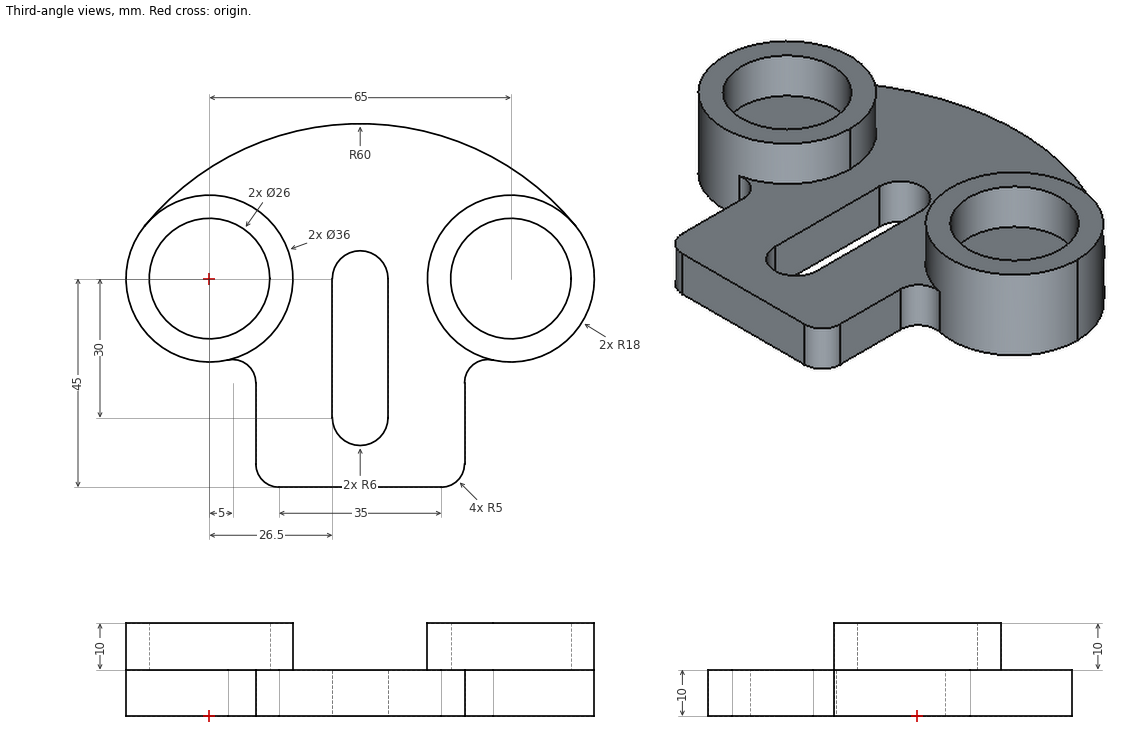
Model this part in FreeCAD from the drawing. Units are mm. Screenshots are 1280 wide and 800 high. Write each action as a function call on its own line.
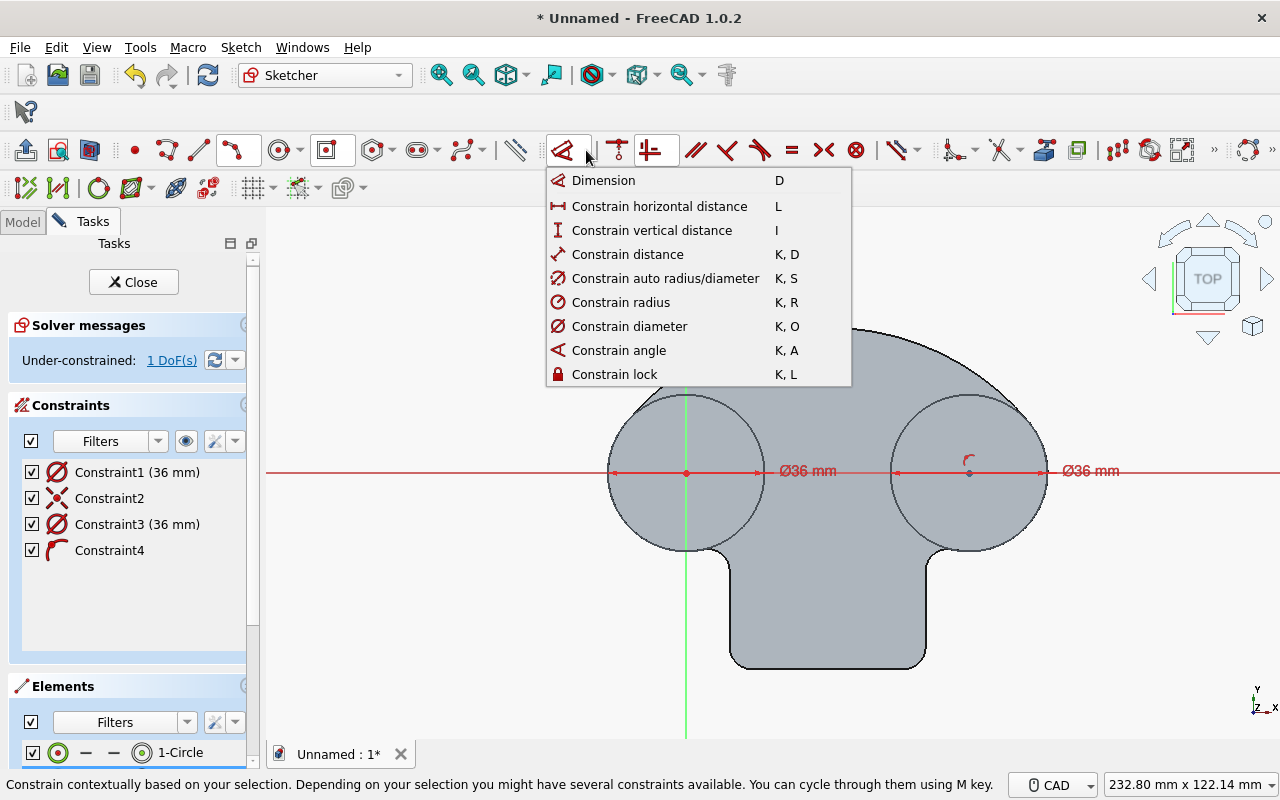
click(699, 206)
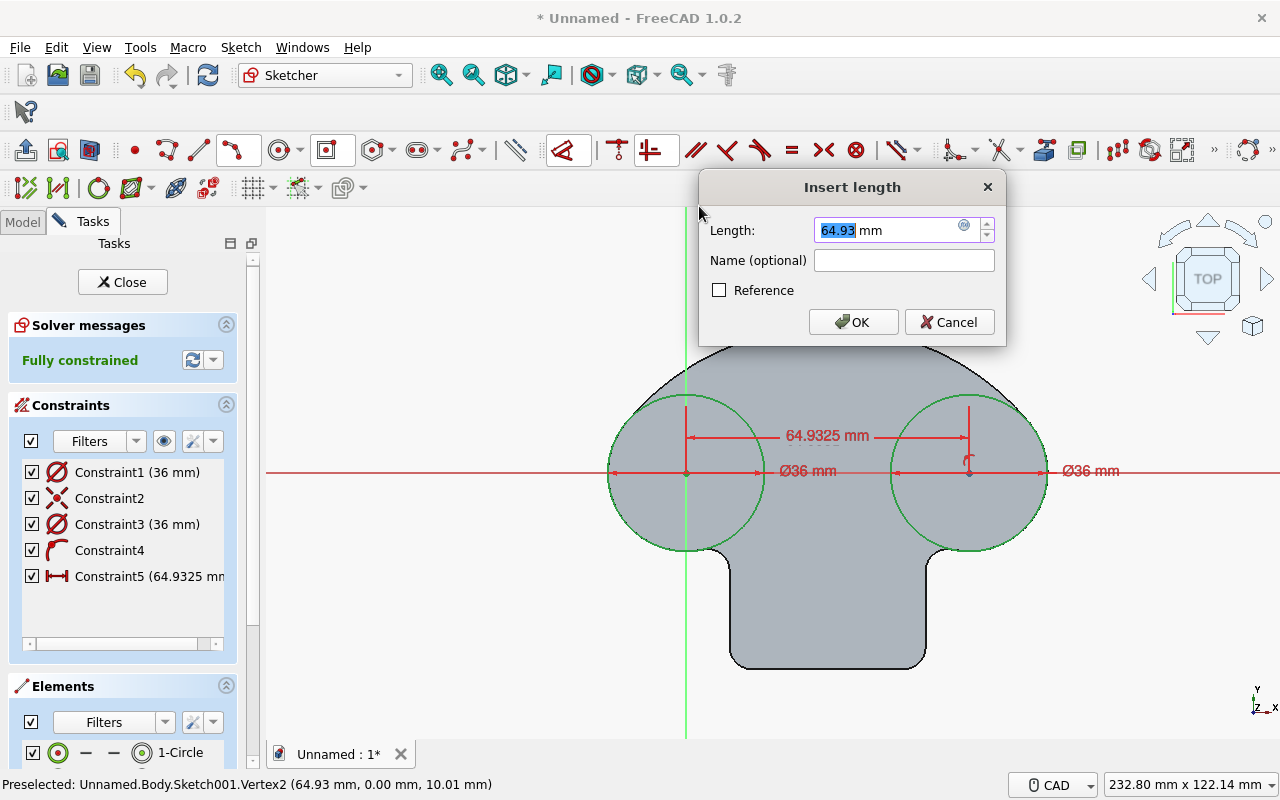
text(65)
key(Return)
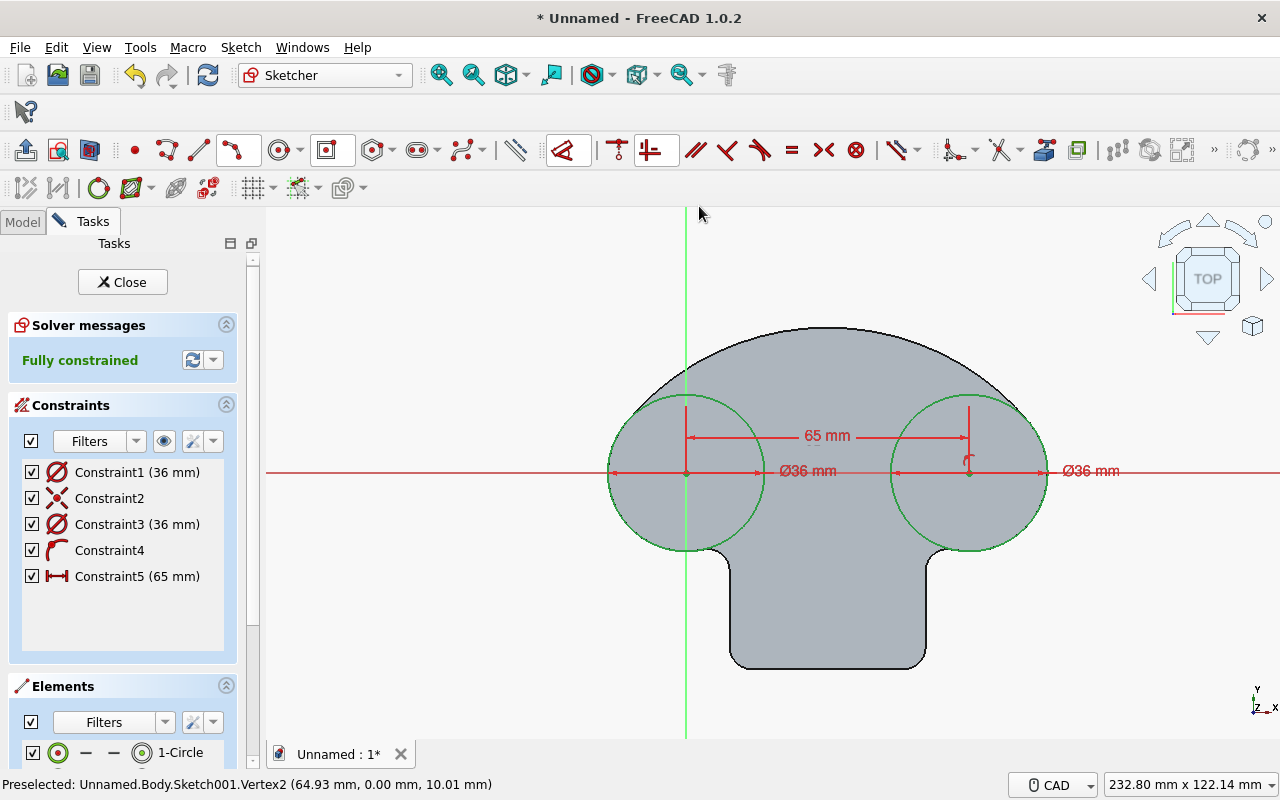
click(123, 282)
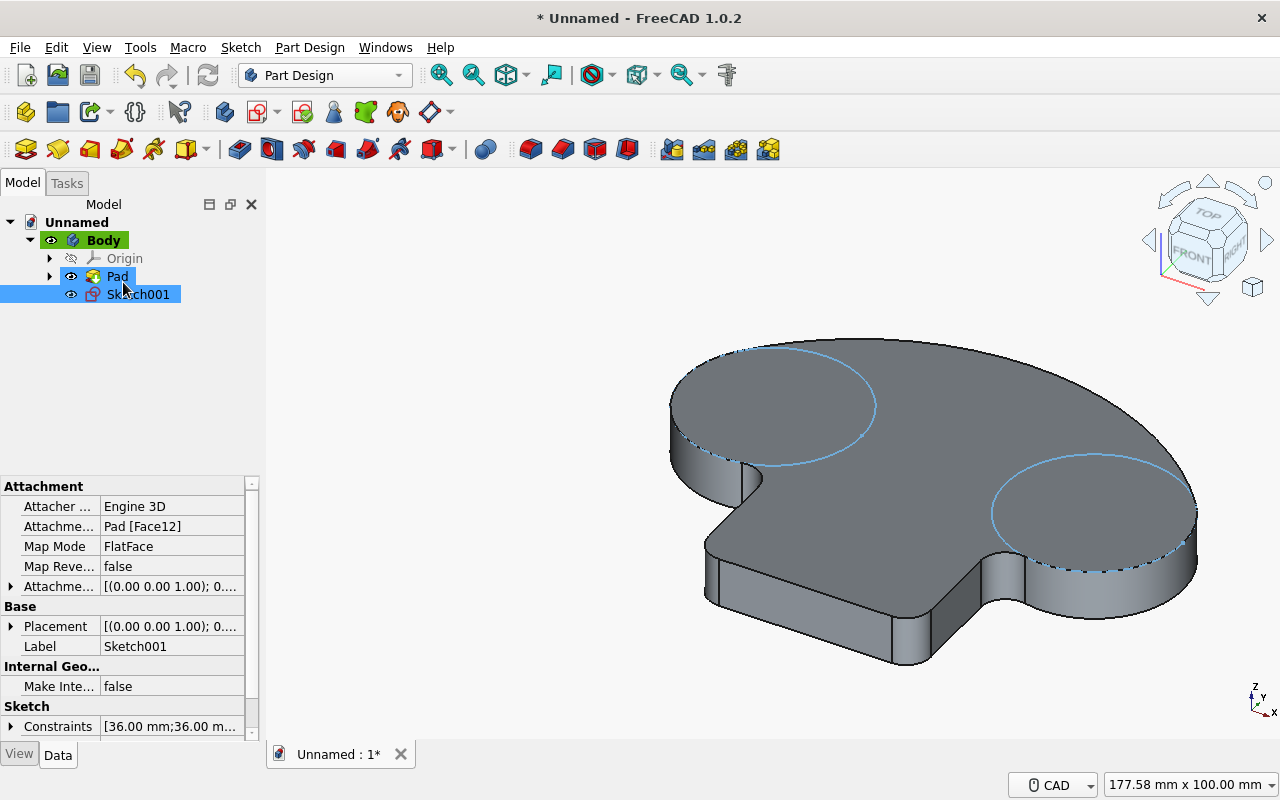
click(26, 150)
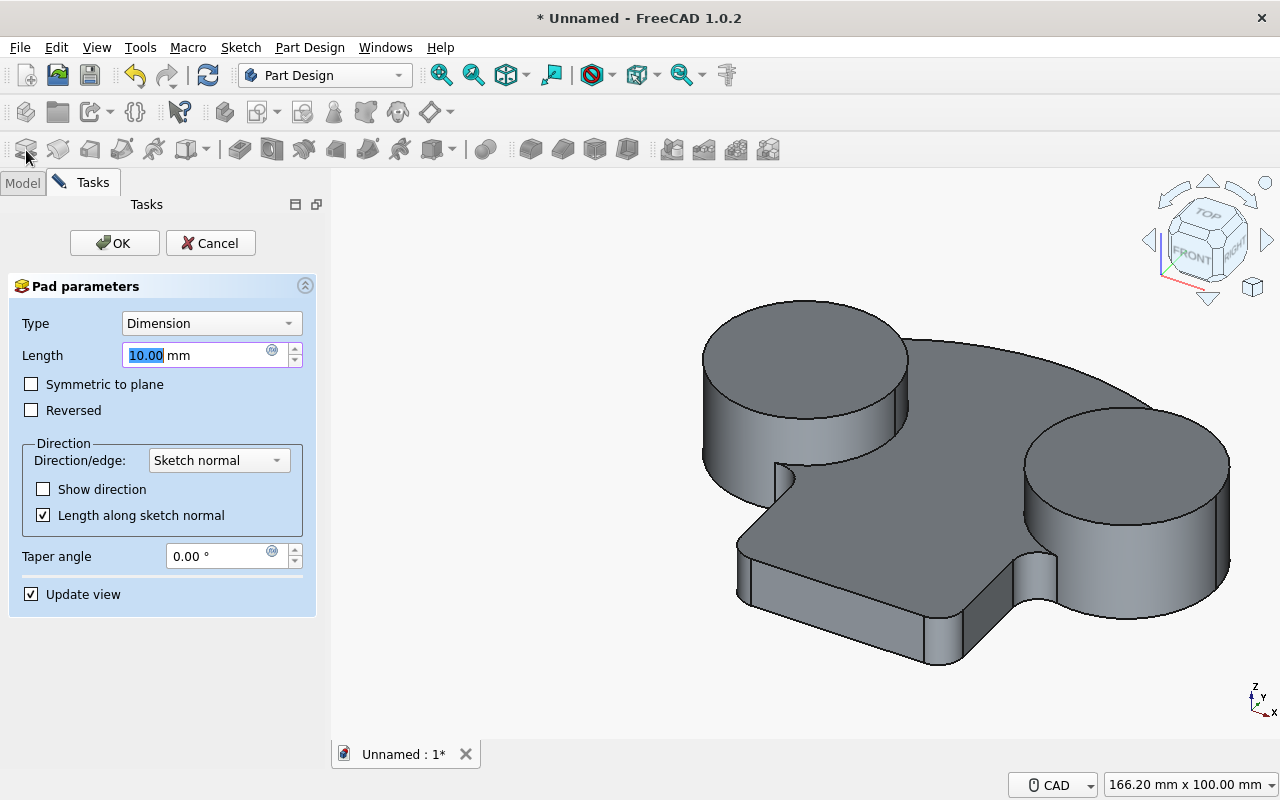
text(10)
key(Tab)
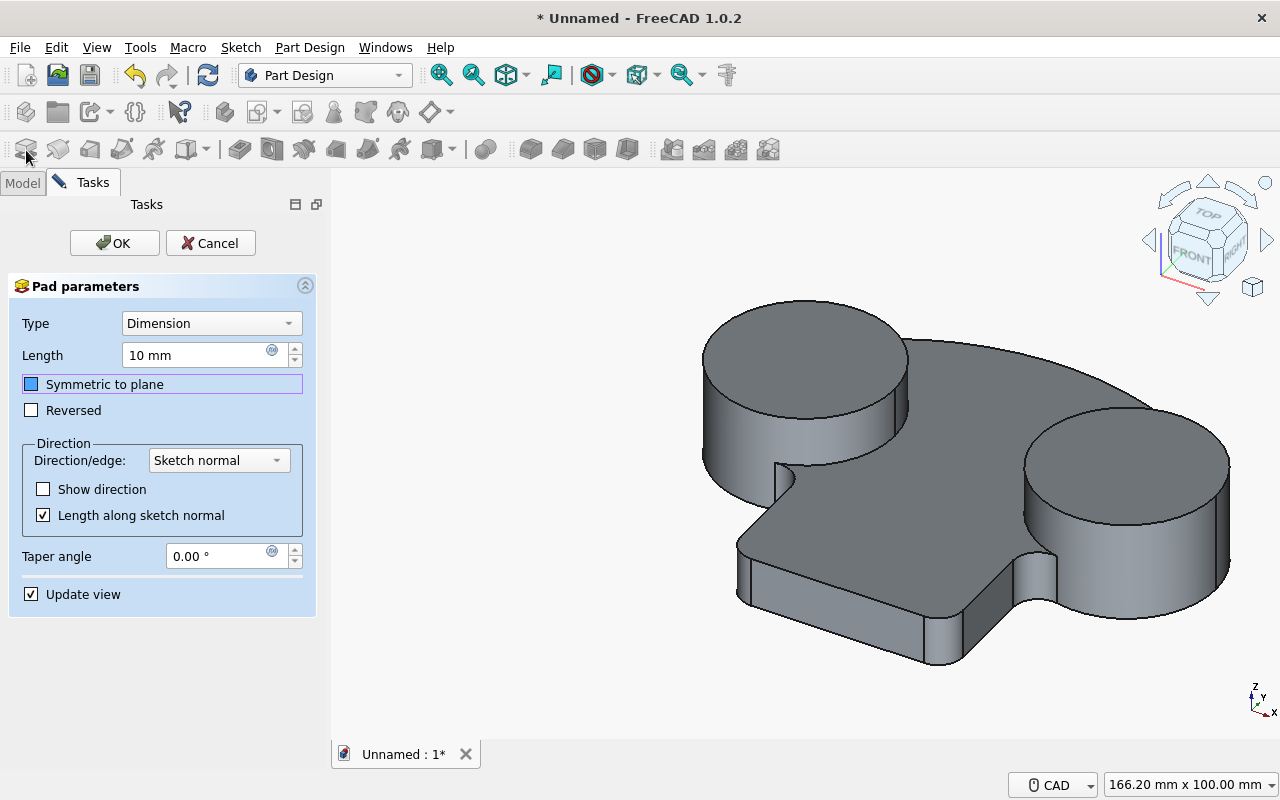
click(115, 243)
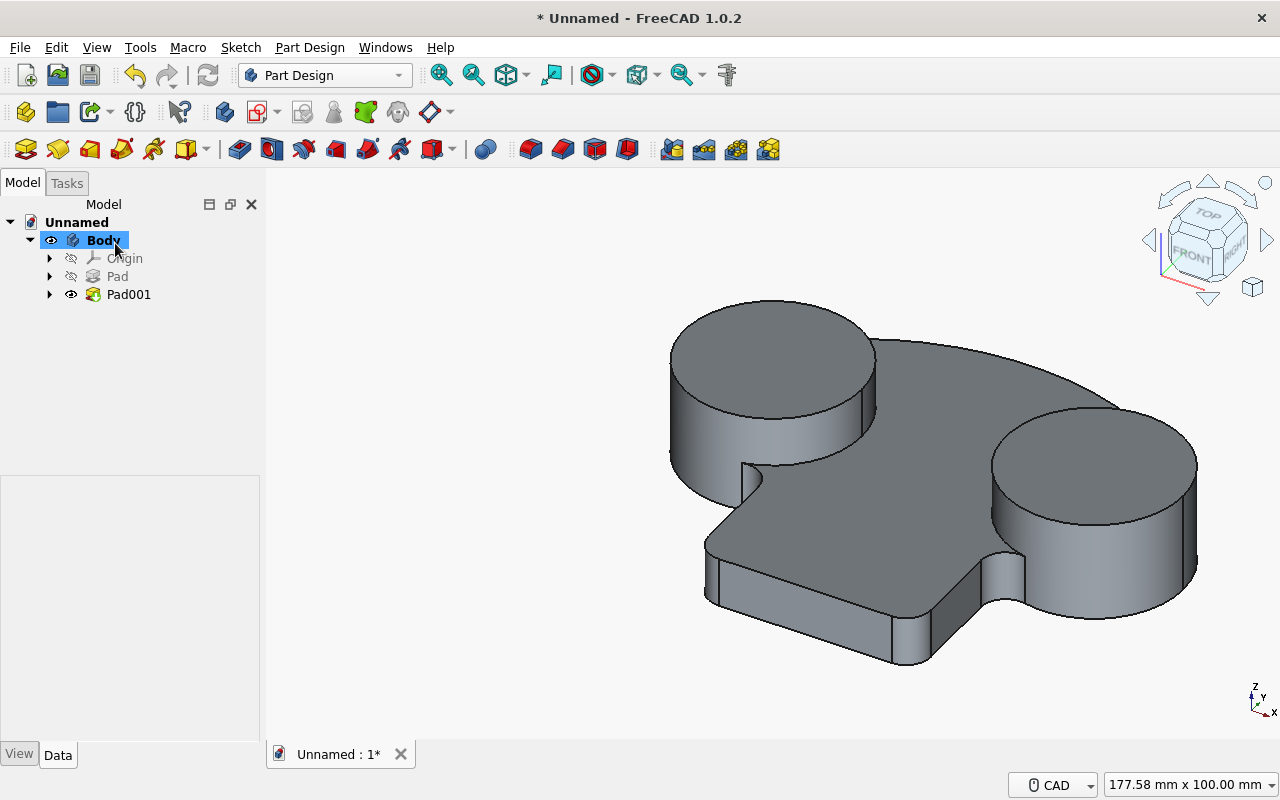
click(1094, 465)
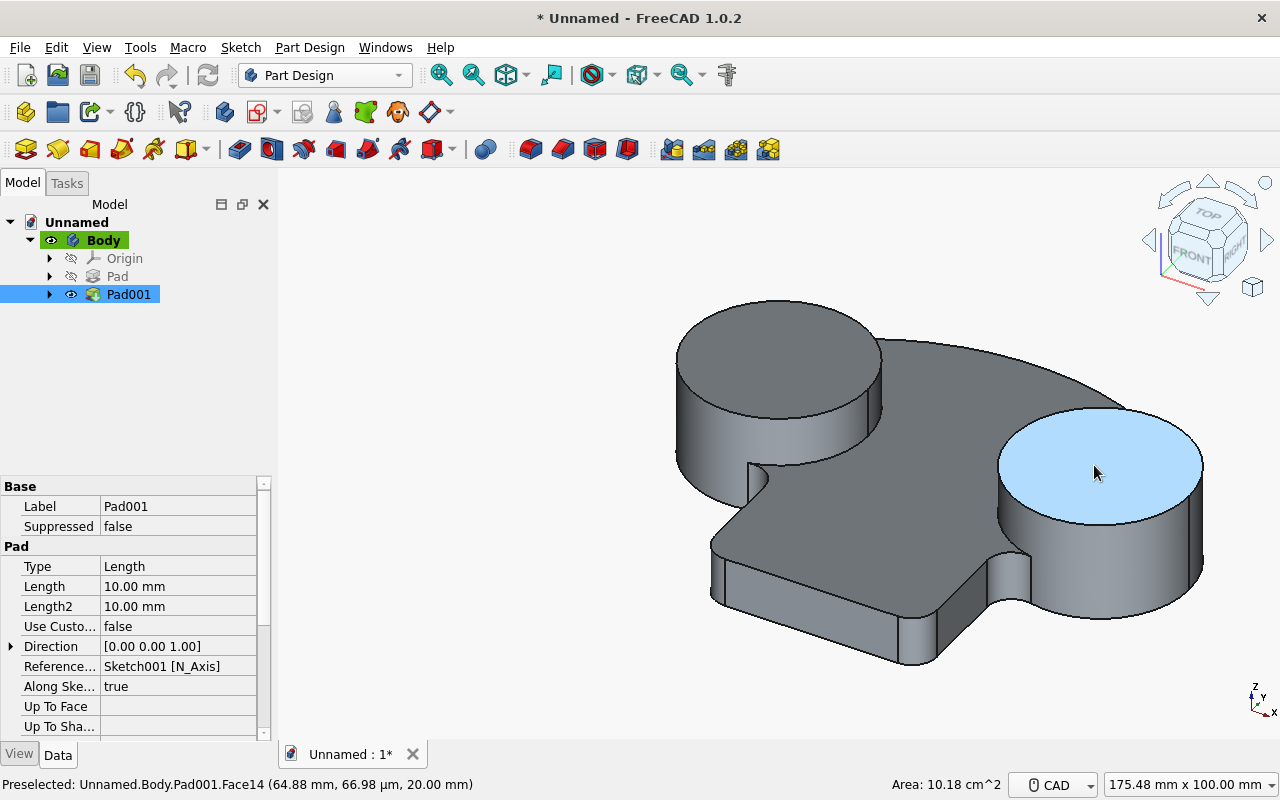
click(258, 112)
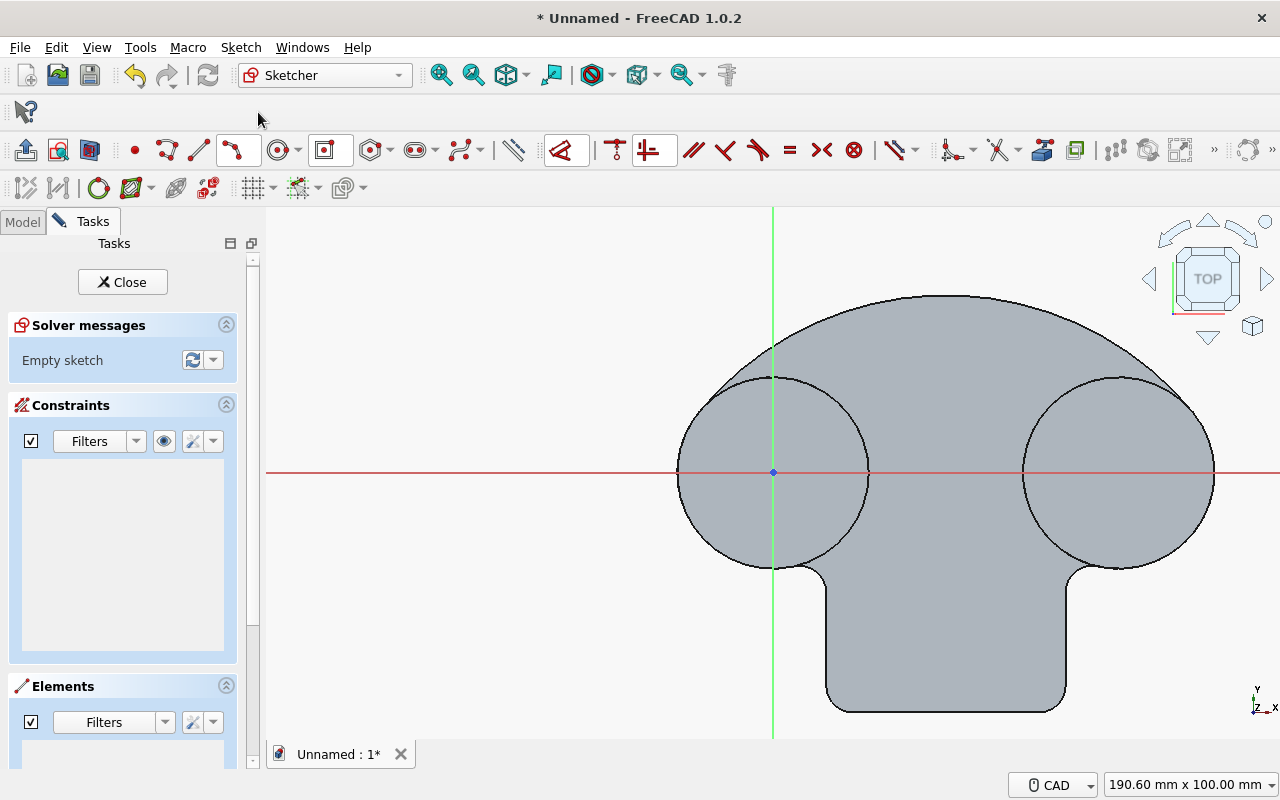
scroll(294, 473, down, 1)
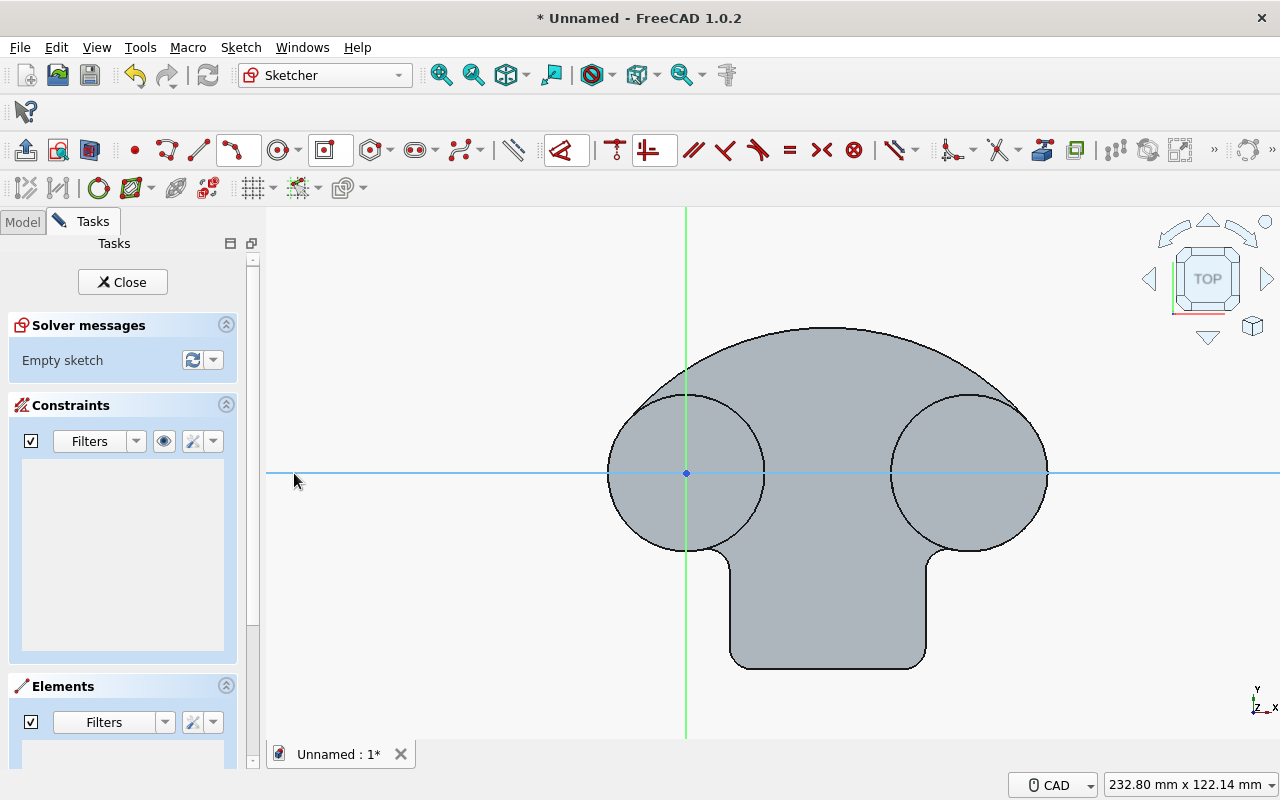
scroll(1078, 473, up, 2)